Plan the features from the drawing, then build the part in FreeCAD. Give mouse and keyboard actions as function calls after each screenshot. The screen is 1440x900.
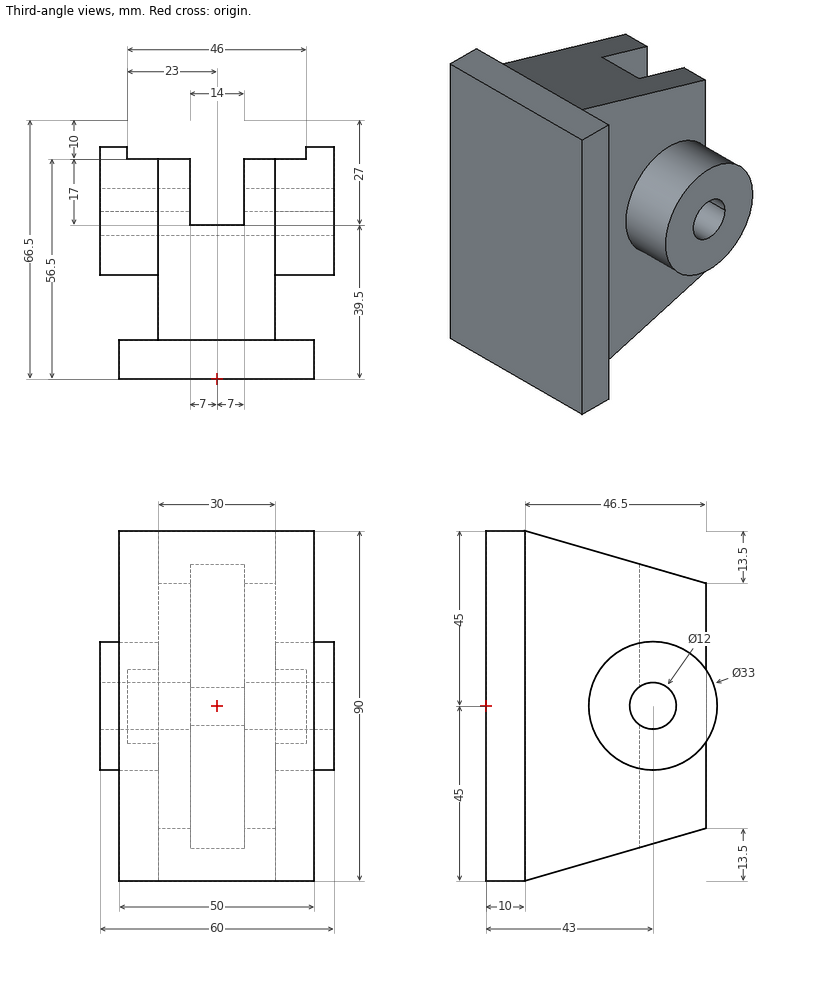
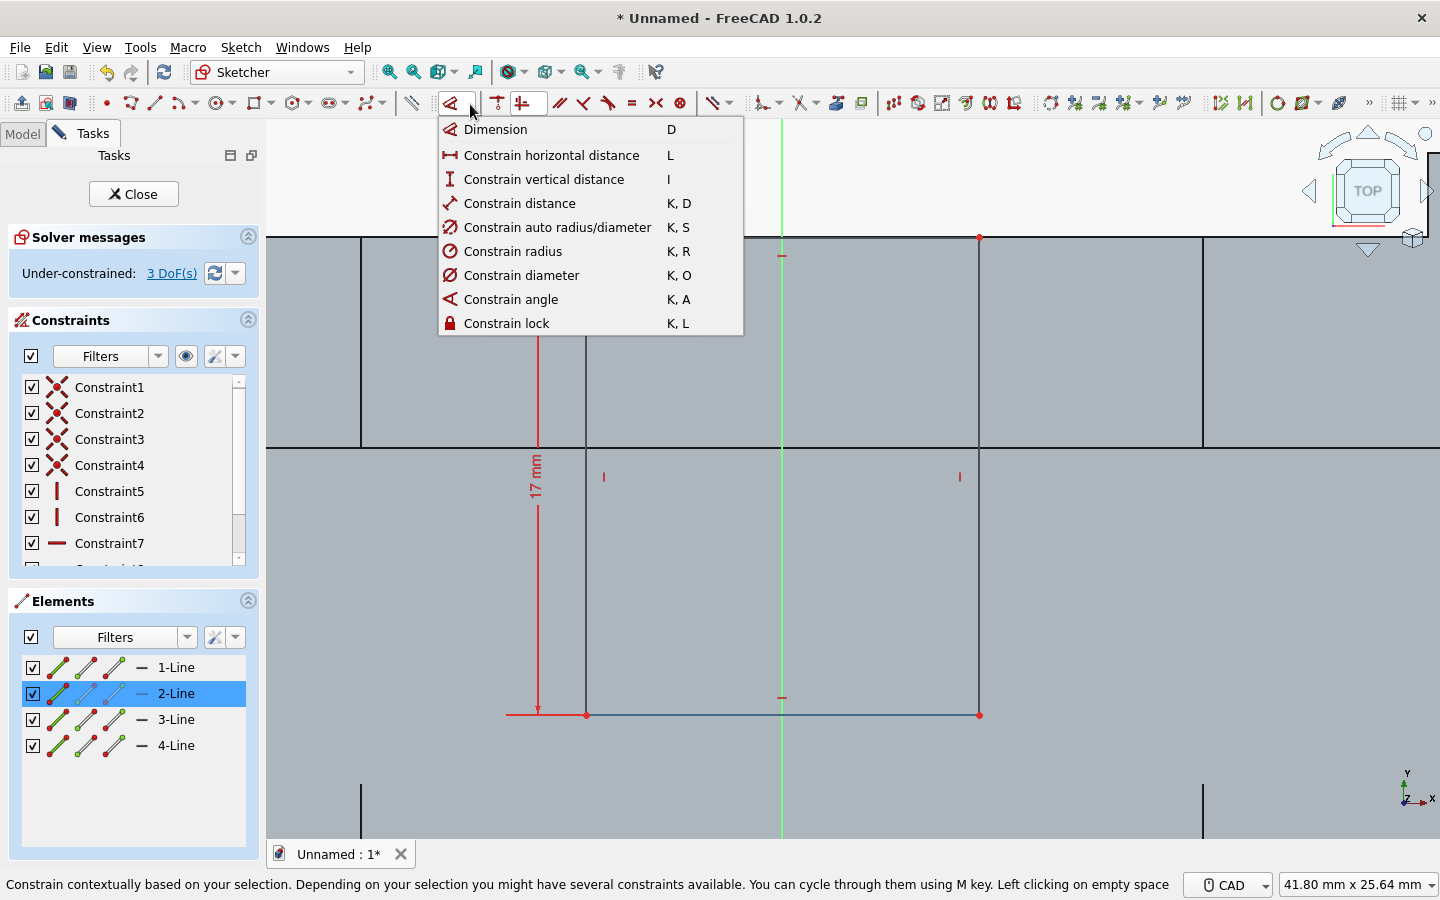
click(591, 155)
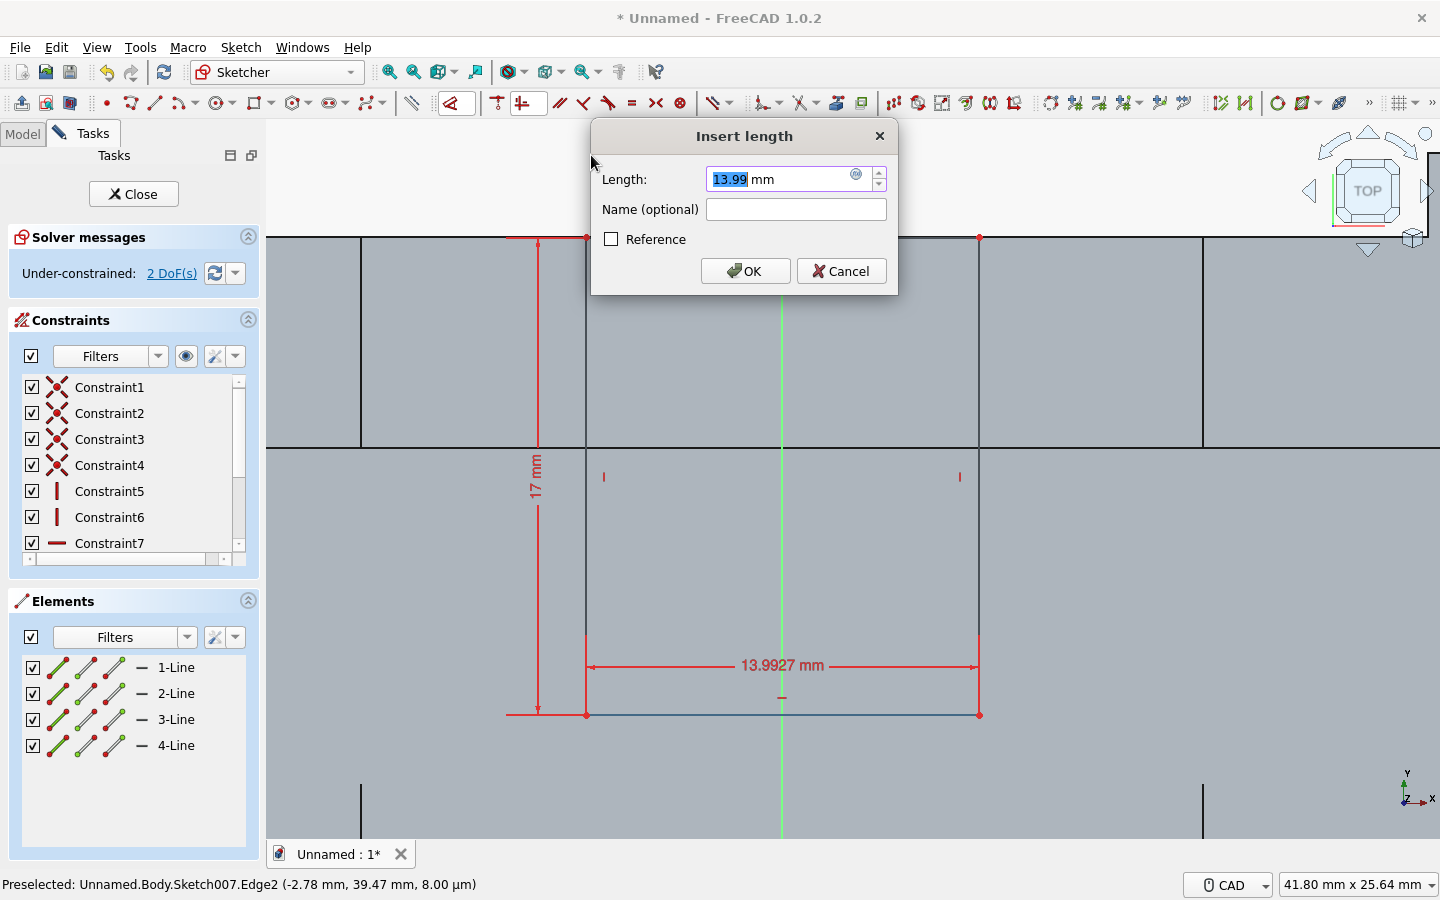
text(14)
key(Return)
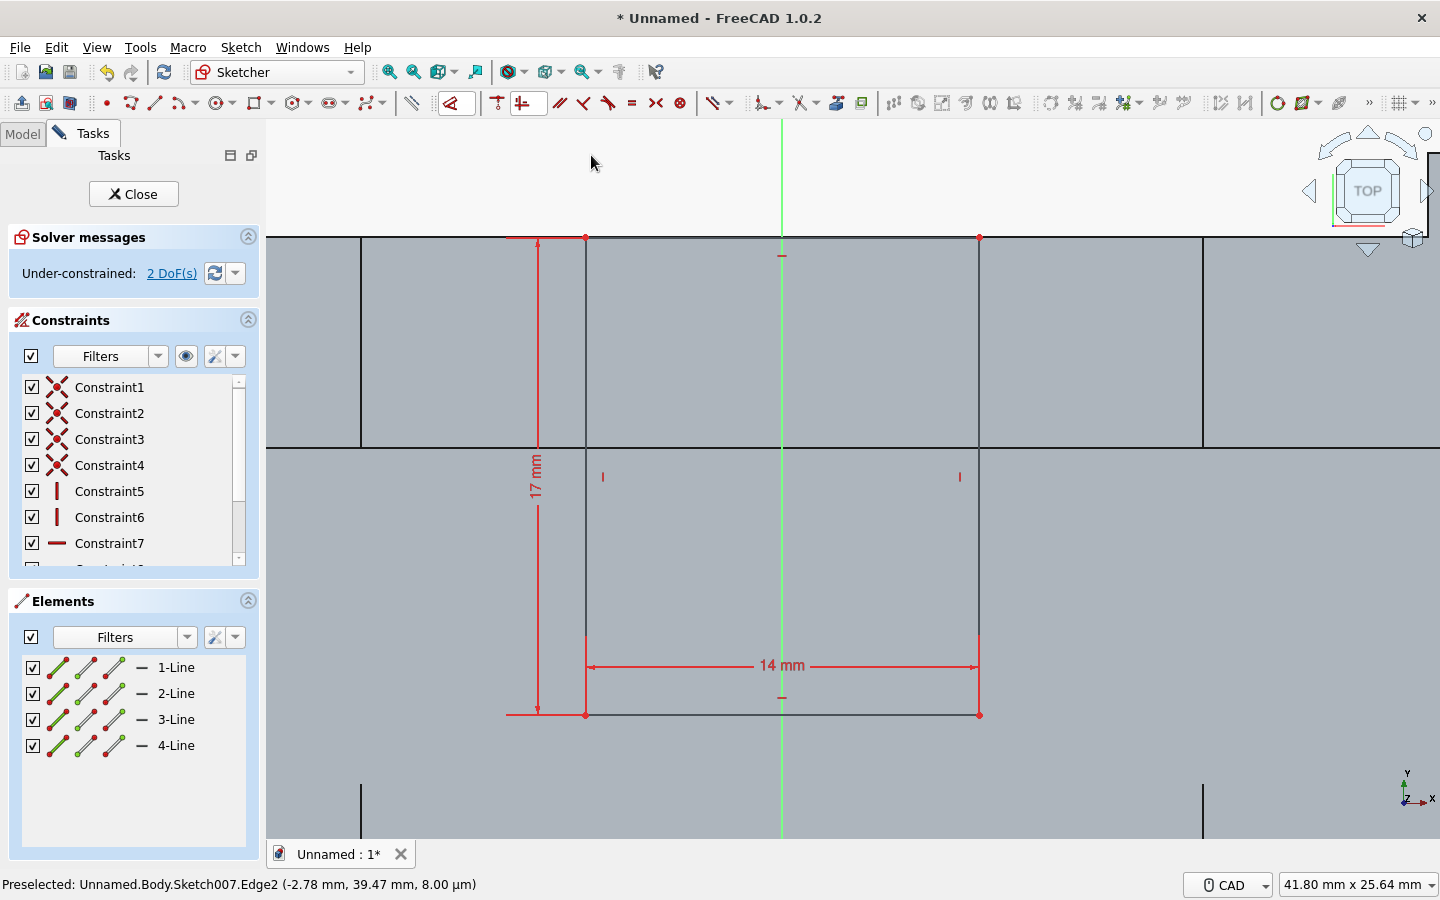
click(586, 238)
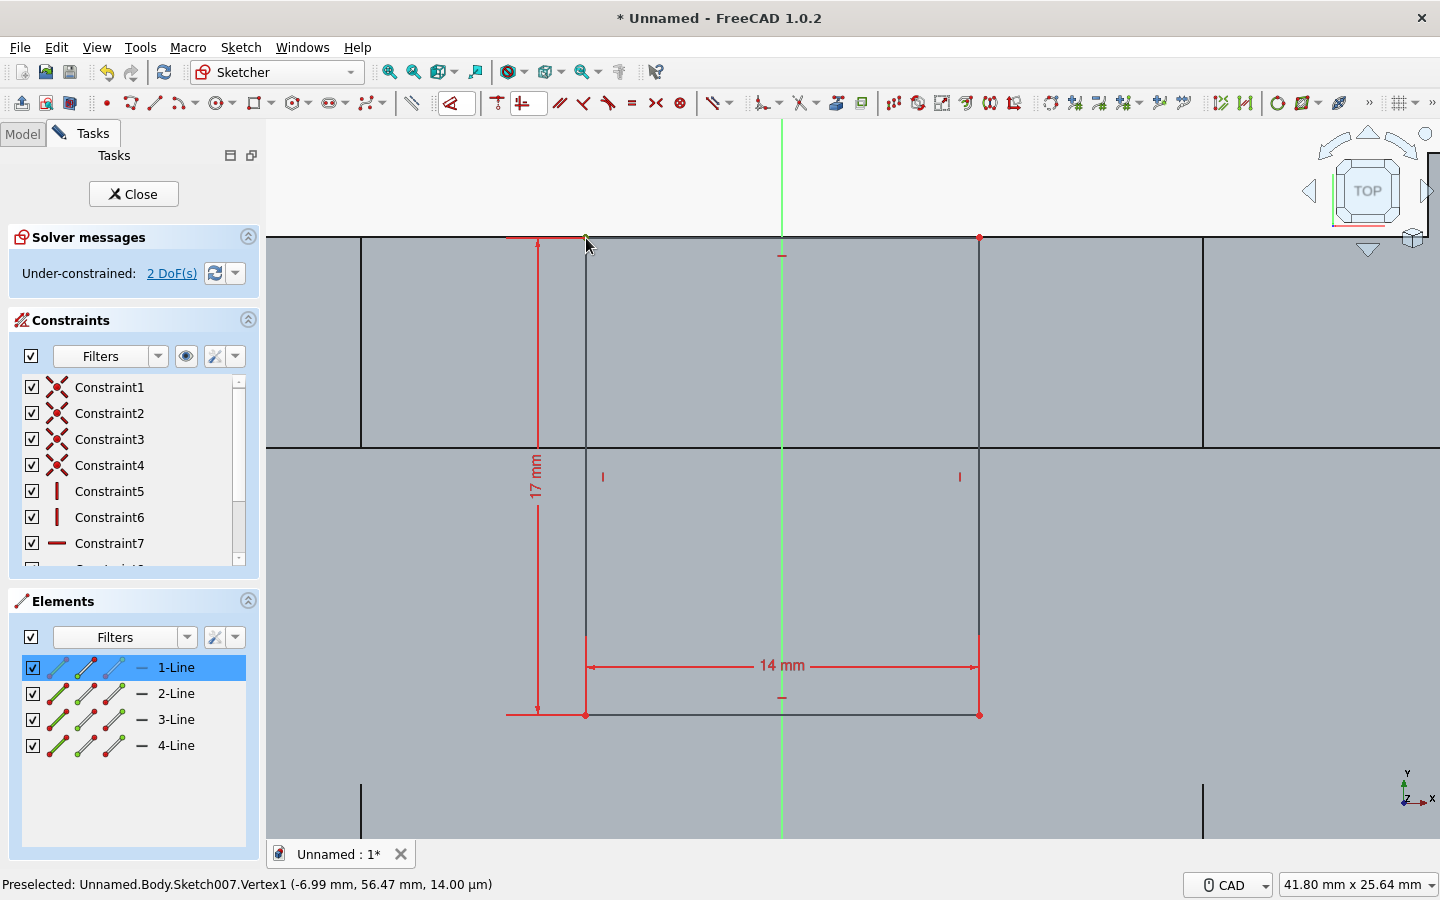
key(l)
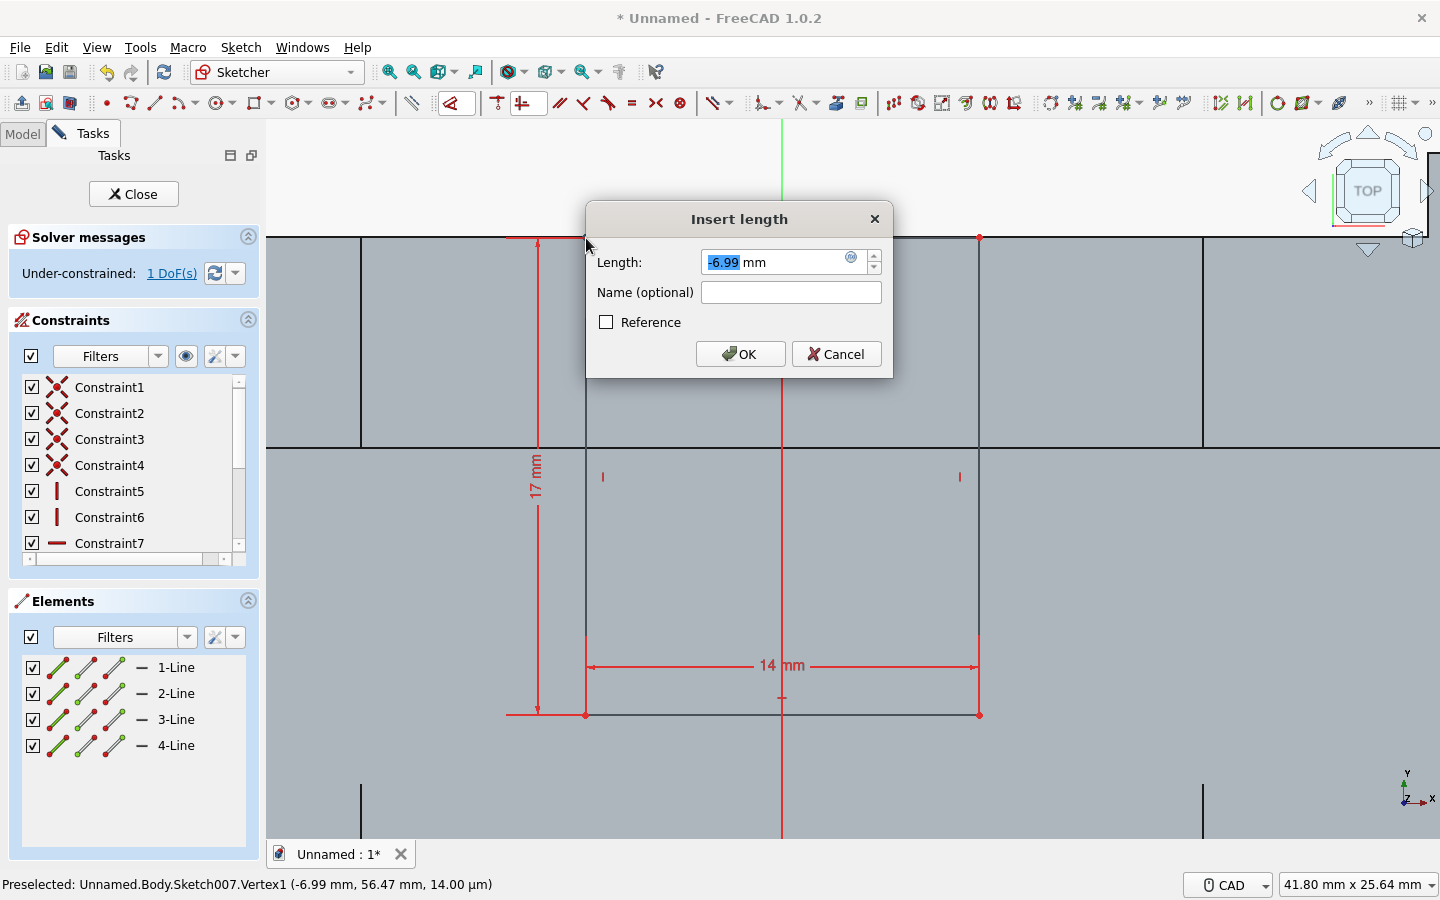
text(-7)
key(Return)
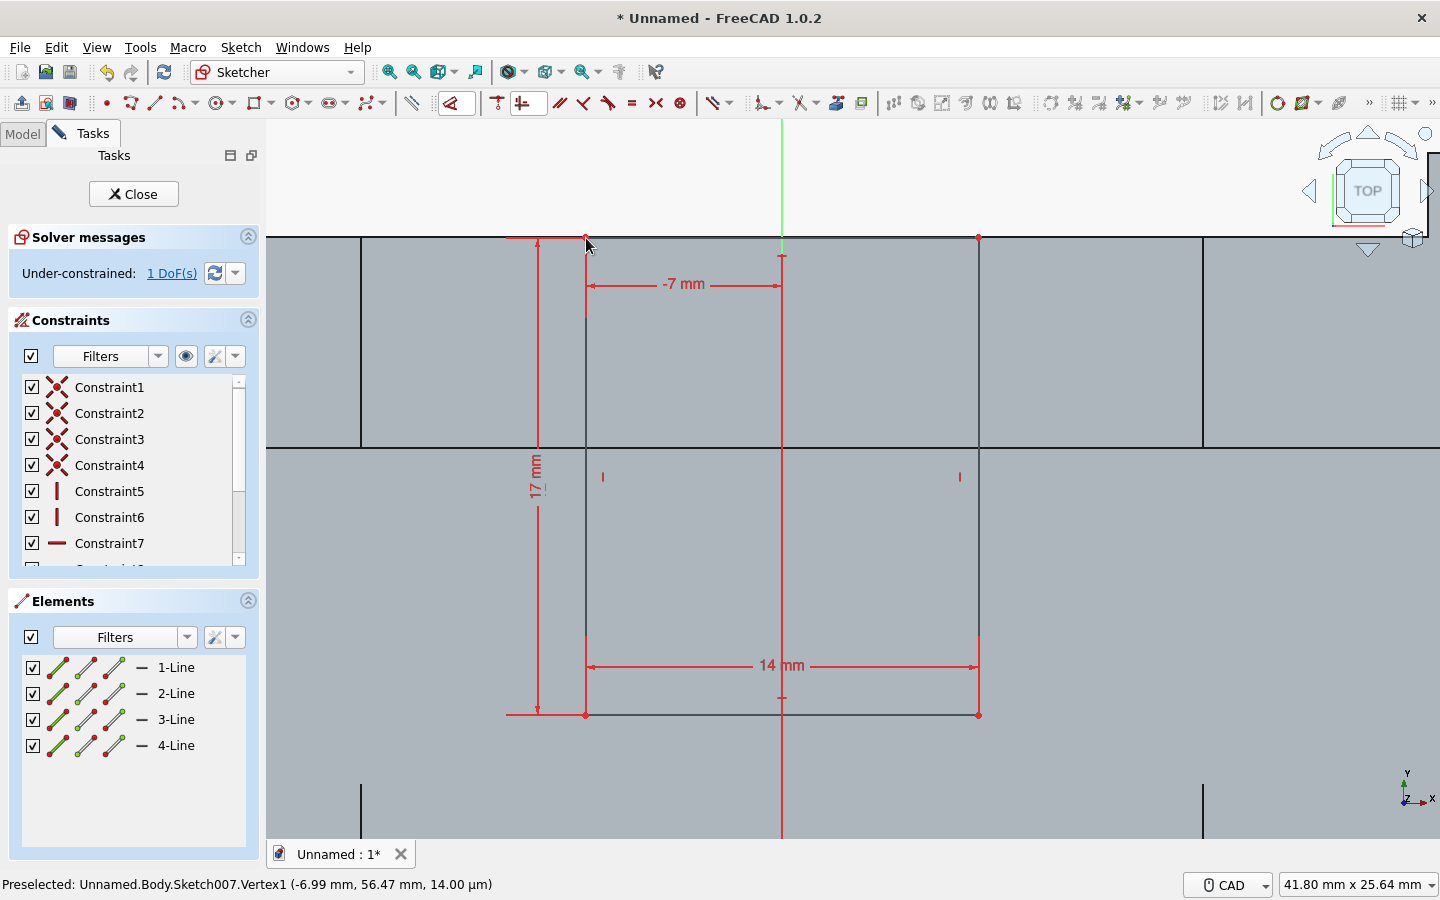
click(586, 238)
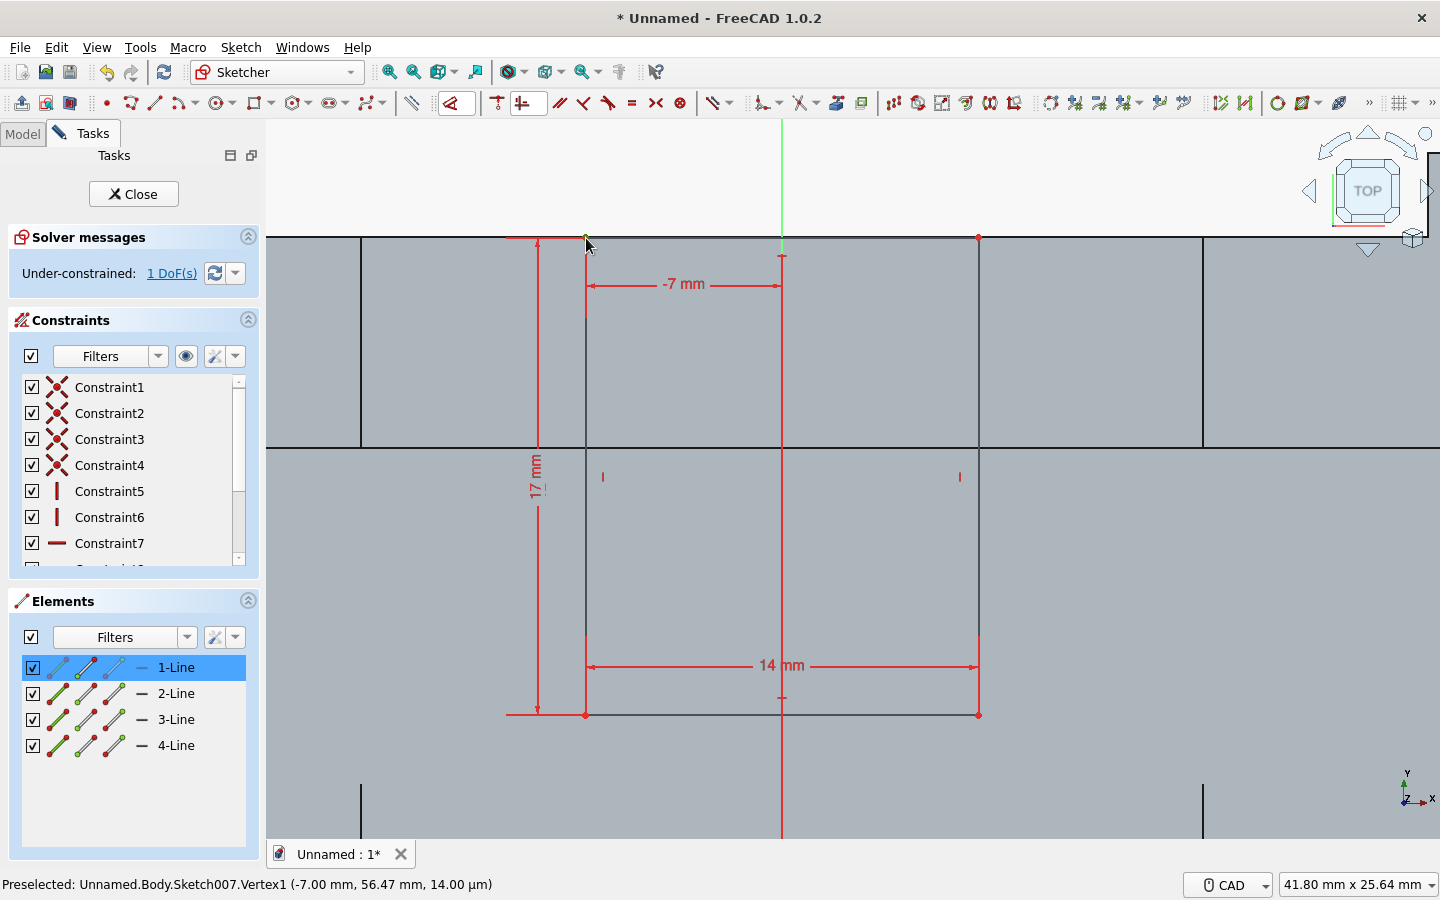
click(470, 104)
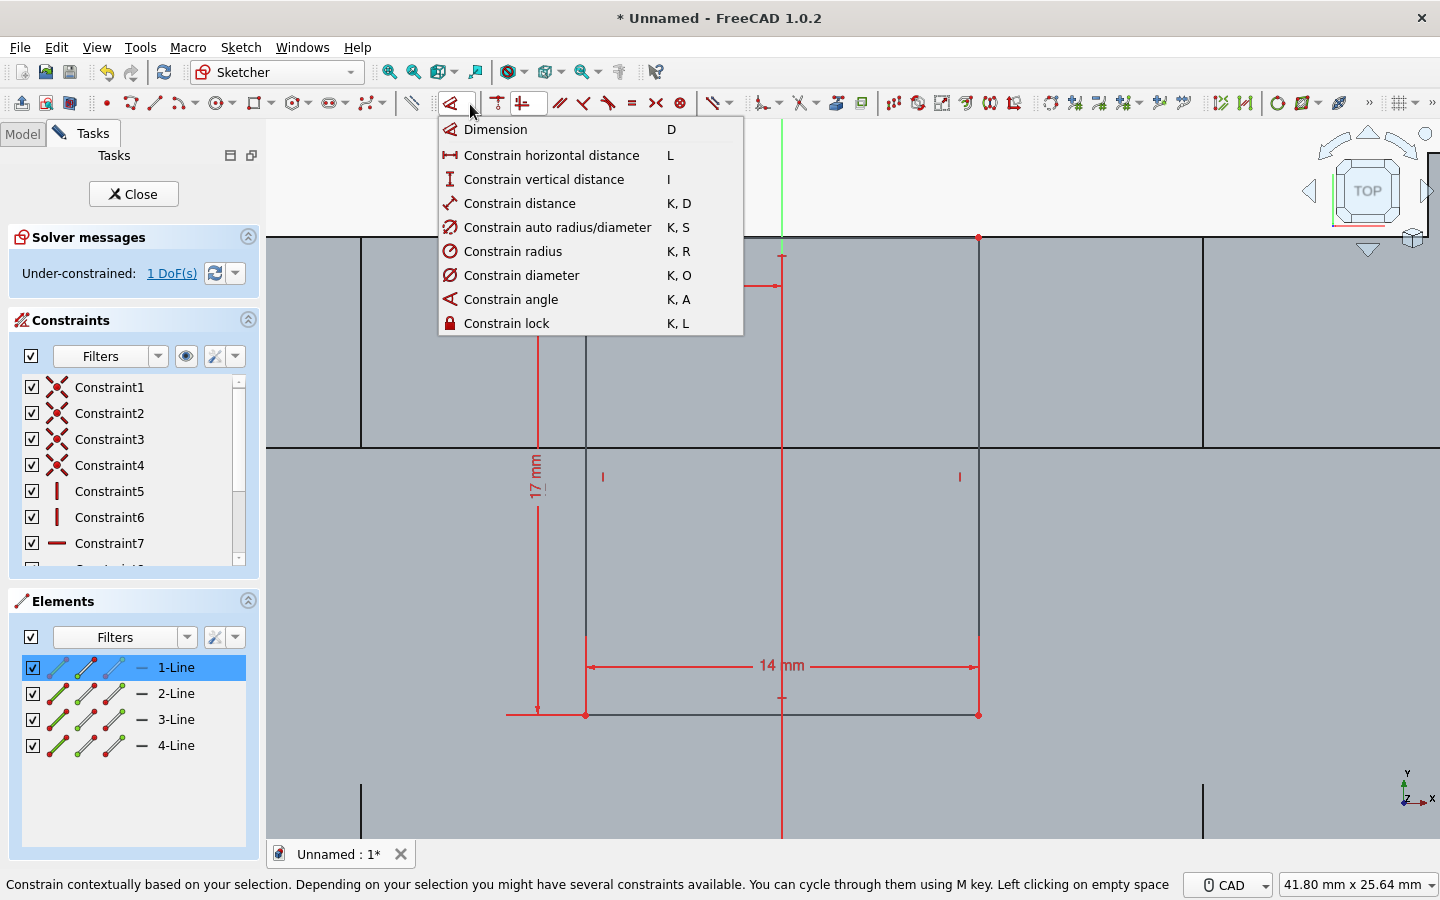
click(591, 179)